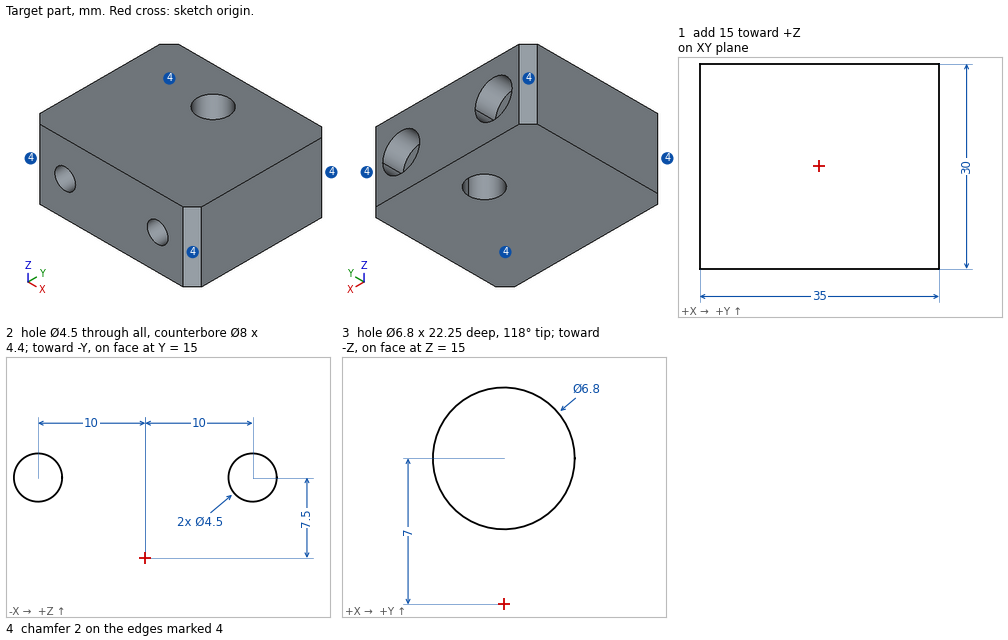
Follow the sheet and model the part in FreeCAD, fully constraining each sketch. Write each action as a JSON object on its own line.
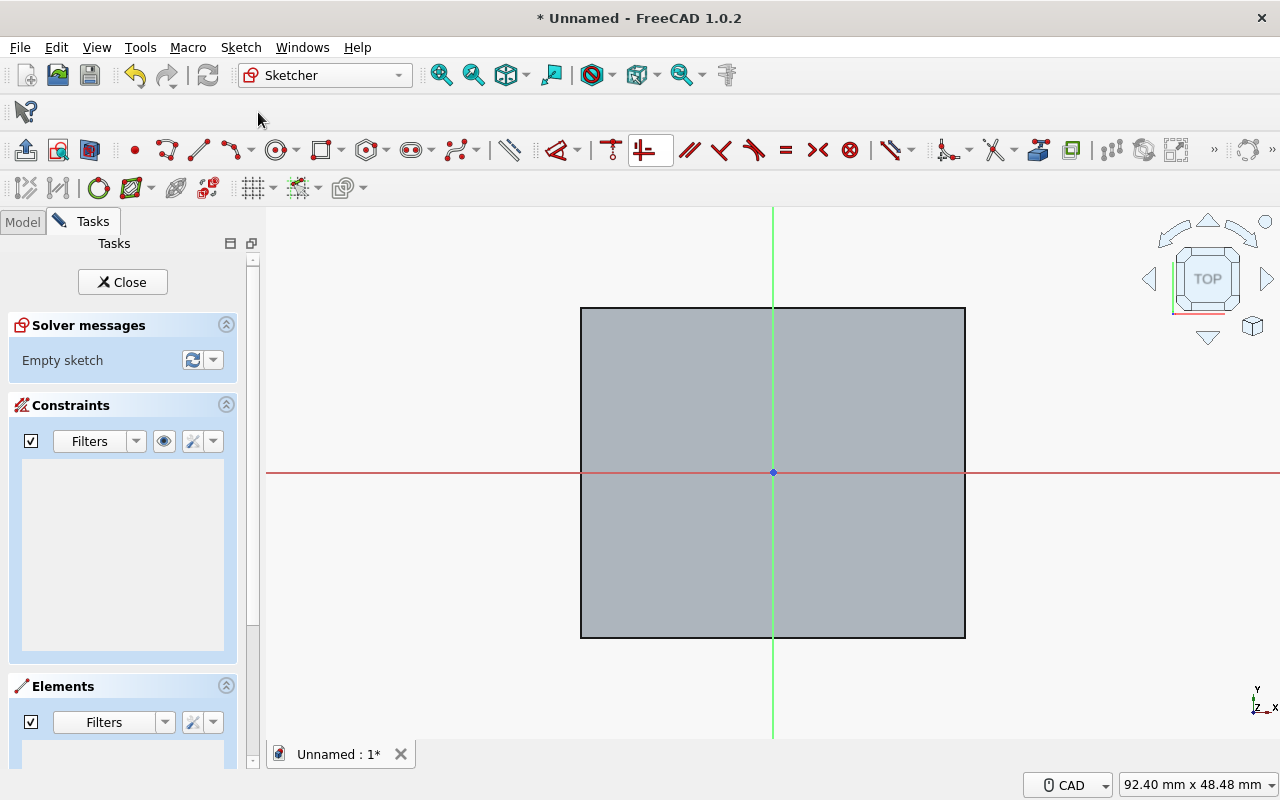
{"action": "scroll", "coordinate": [813, 383], "scroll_direction": "up", "scroll_amount": 5}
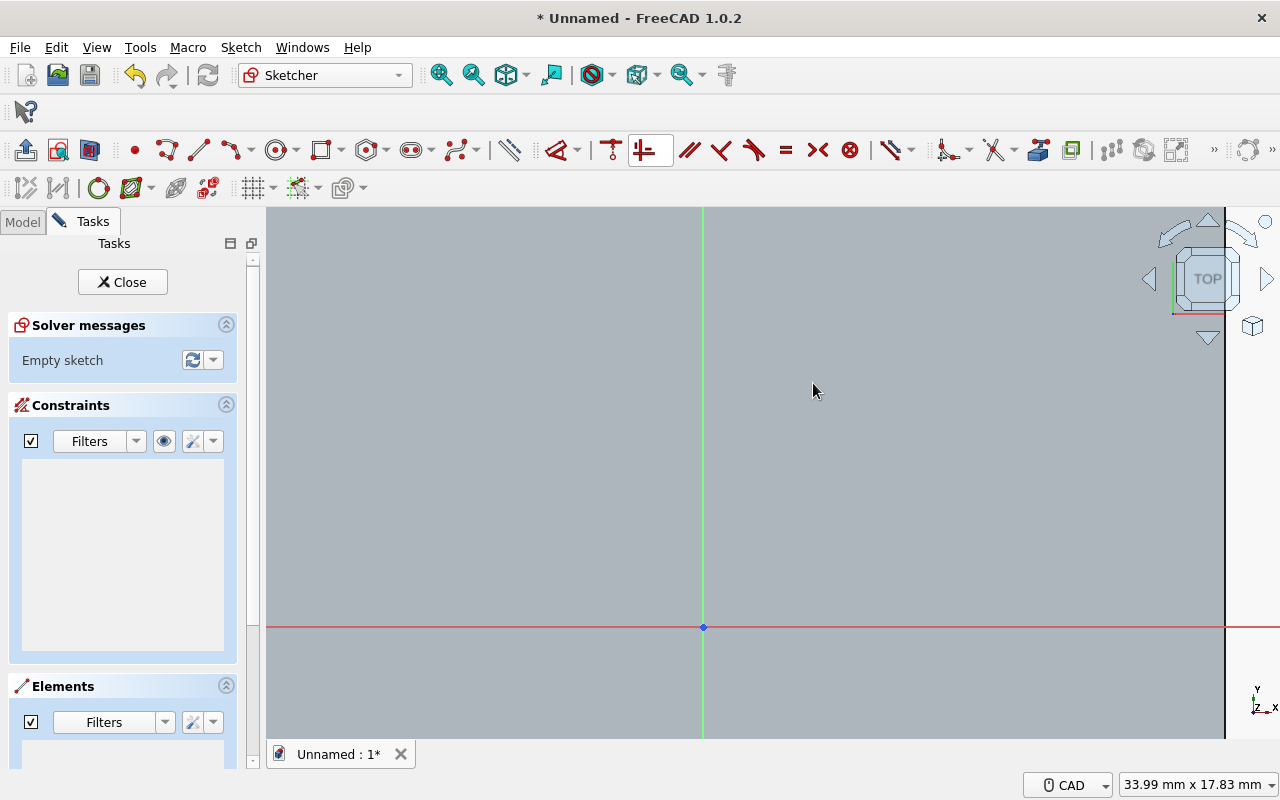
{"action": "key", "text": "g c"}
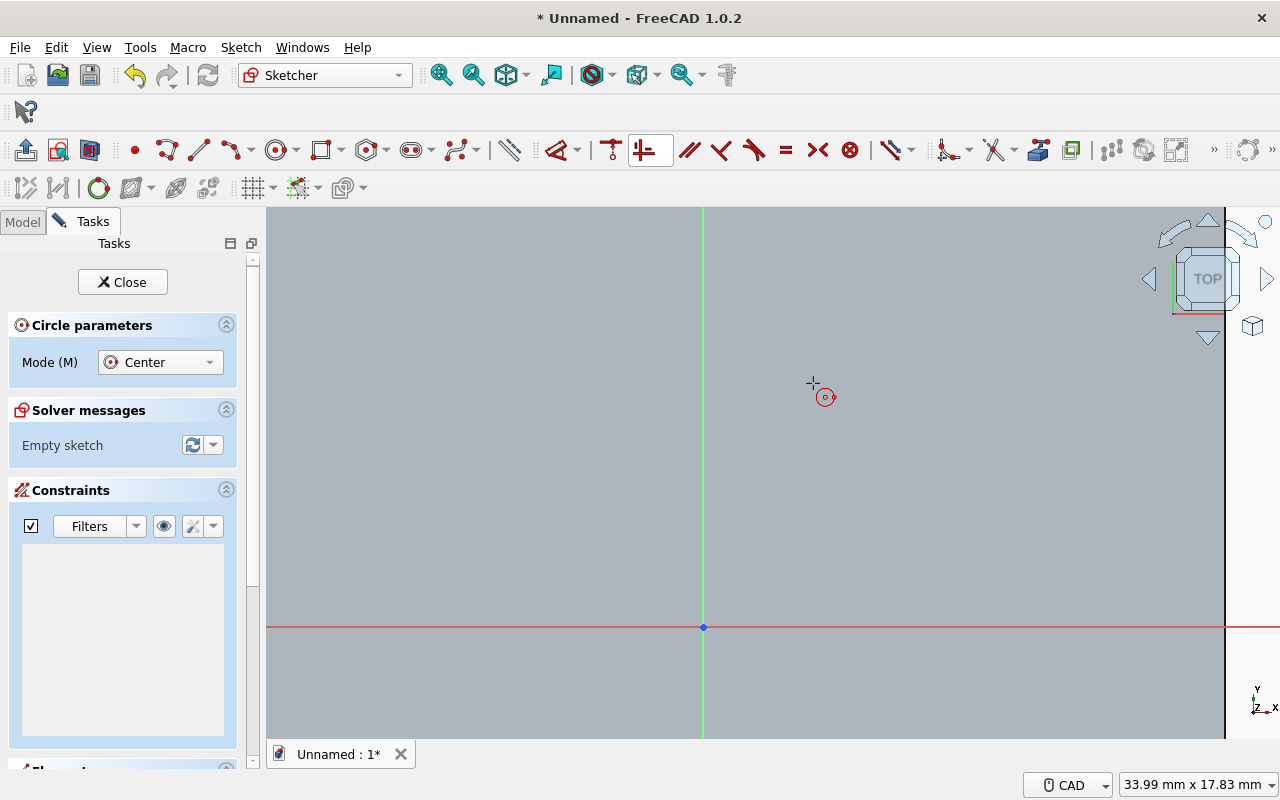
{"action": "left_click", "coordinate": [703, 418]}
{"action": "mouse_move", "coordinate": [775, 347]}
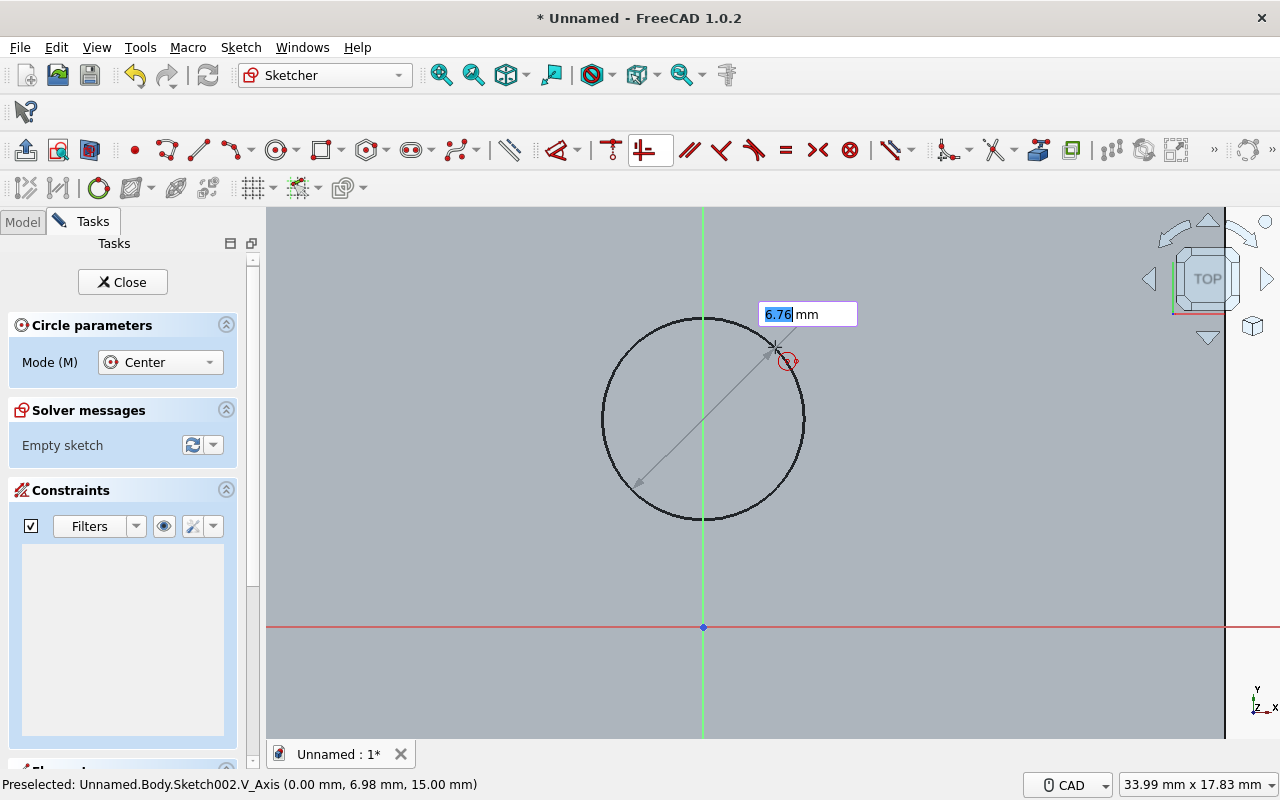
{"action": "type", "text": "6.8"}
{"action": "key", "text": "Return"}
{"action": "key", "text": "Escape"}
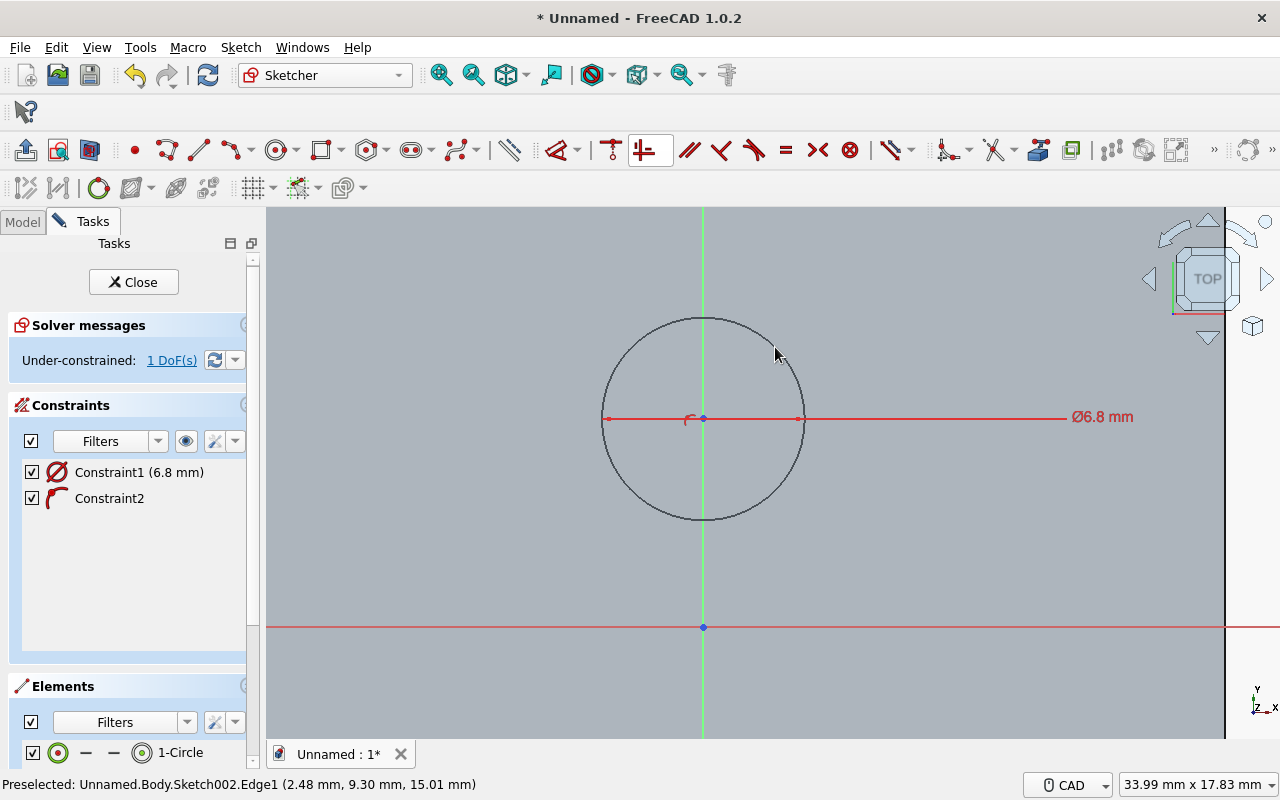
{"action": "left_click", "coordinate": [556, 150]}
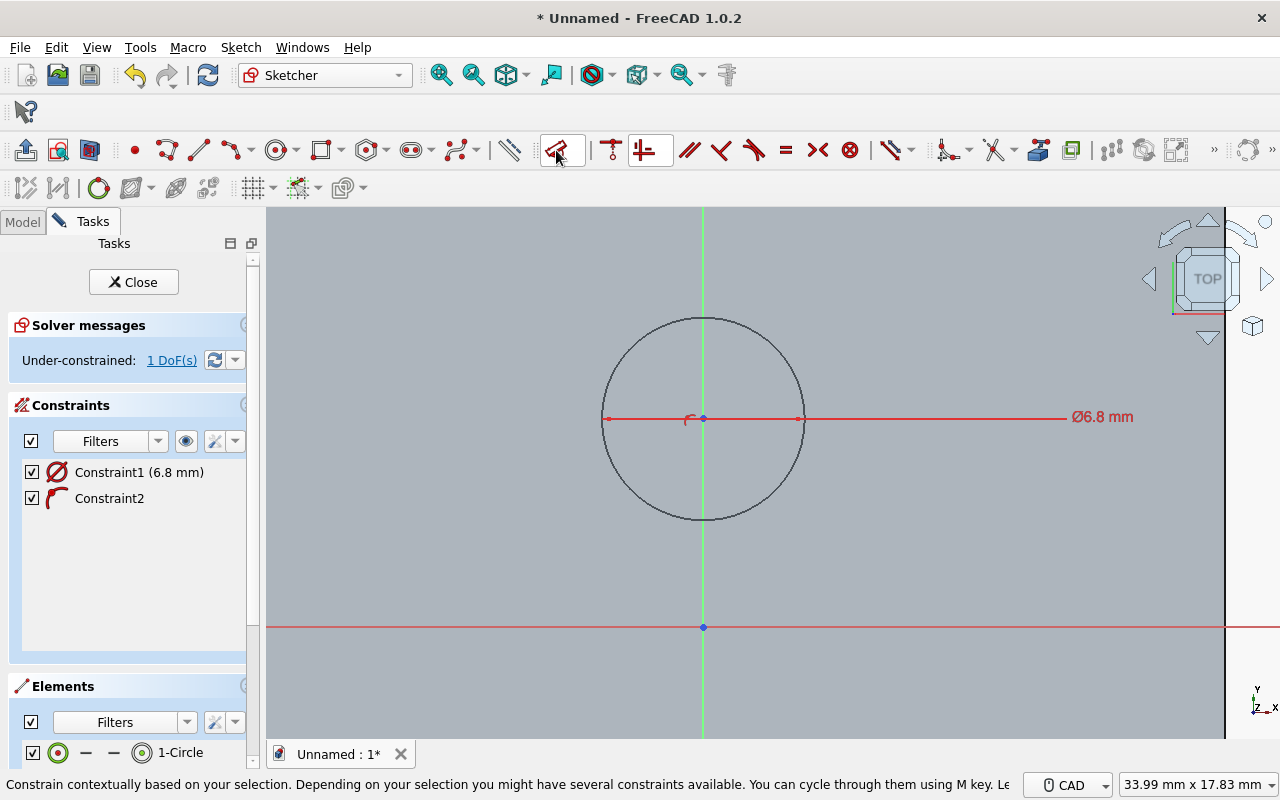
{"action": "left_click", "coordinate": [703, 419]}
{"action": "left_click", "coordinate": [737, 475]}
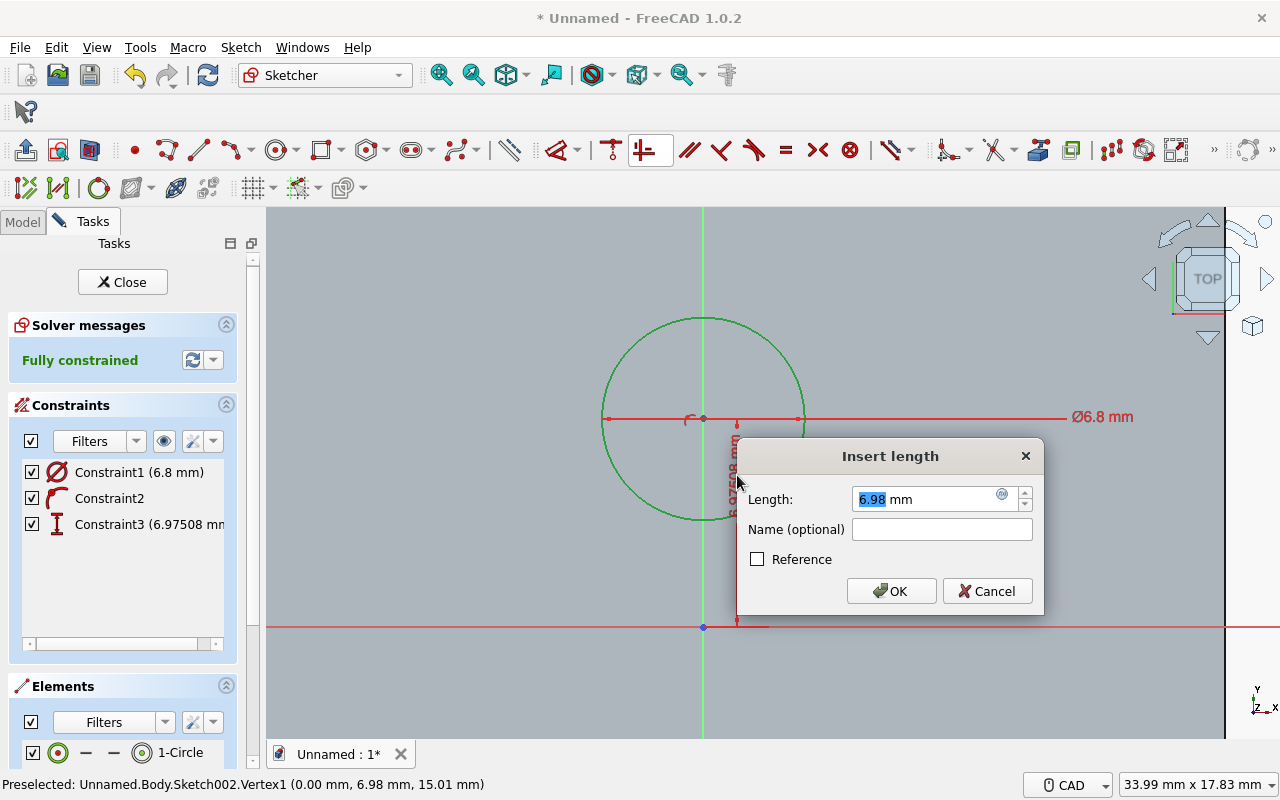
{"action": "type", "text": "7"}
{"action": "key", "text": "Return"}
{"action": "key", "text": "Escape"}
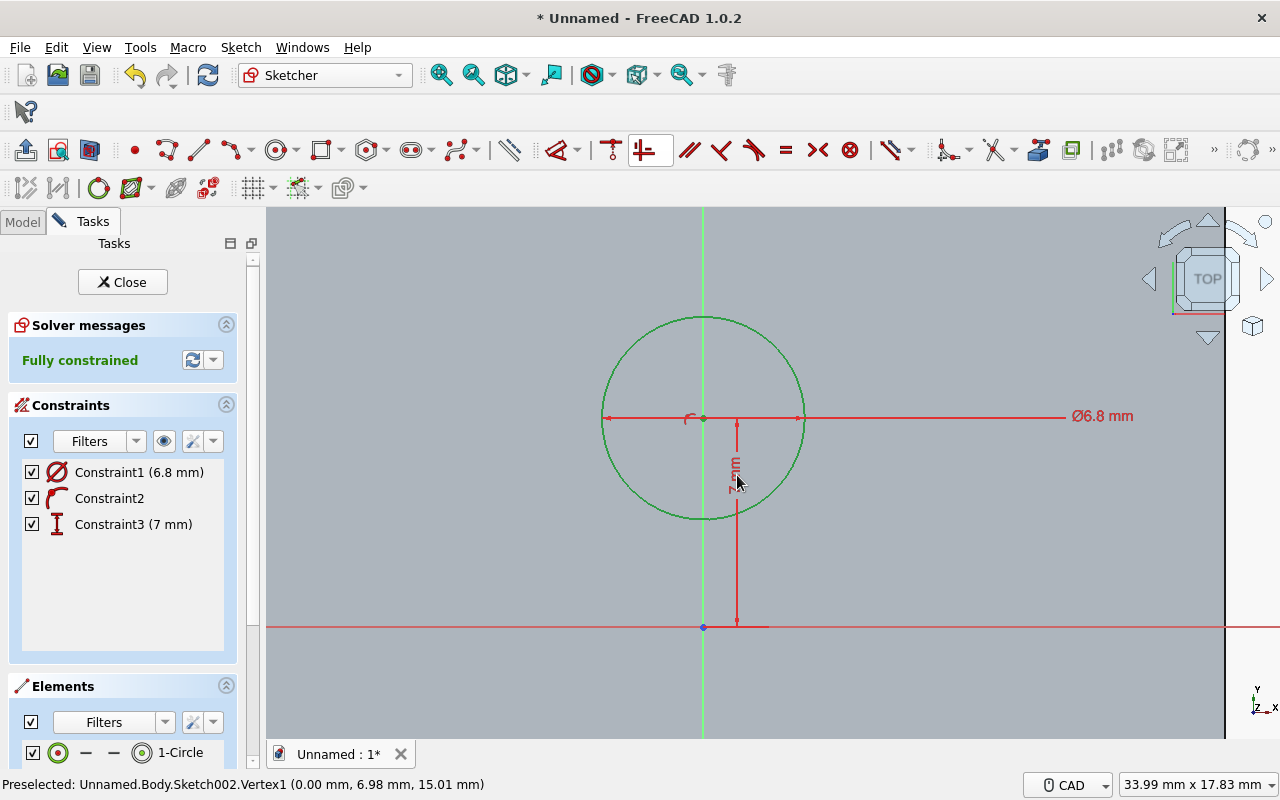
{"action": "left_click", "coordinate": [123, 282]}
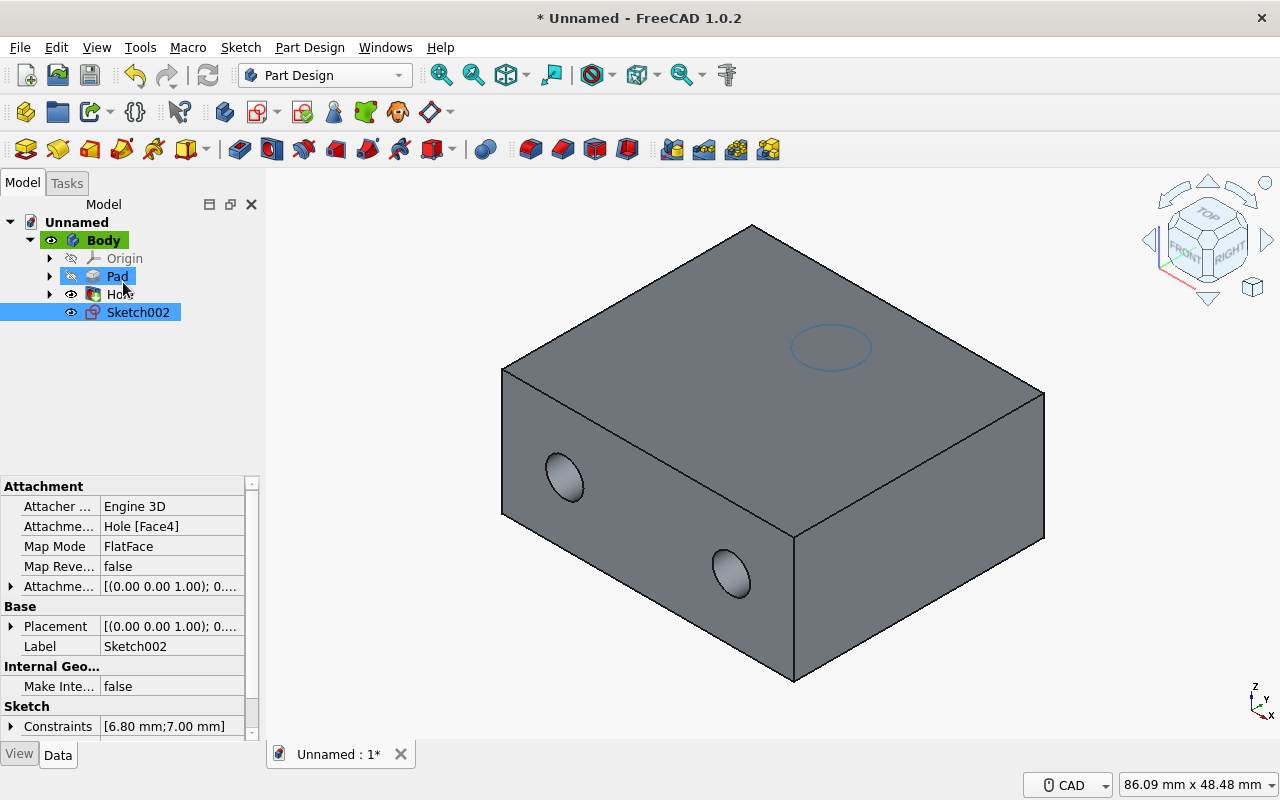
{"action": "left_click", "coordinate": [272, 150]}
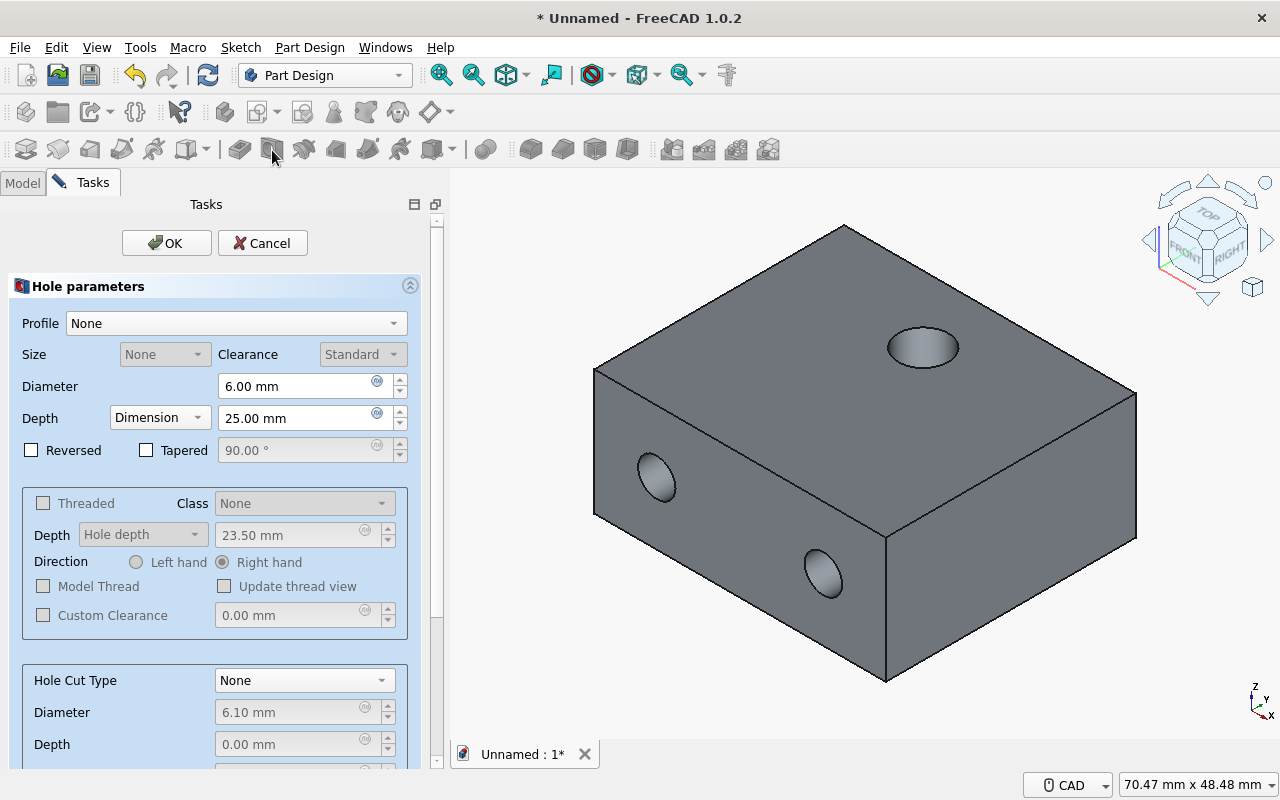
{"action": "triple_click", "coordinate": [305, 386]}